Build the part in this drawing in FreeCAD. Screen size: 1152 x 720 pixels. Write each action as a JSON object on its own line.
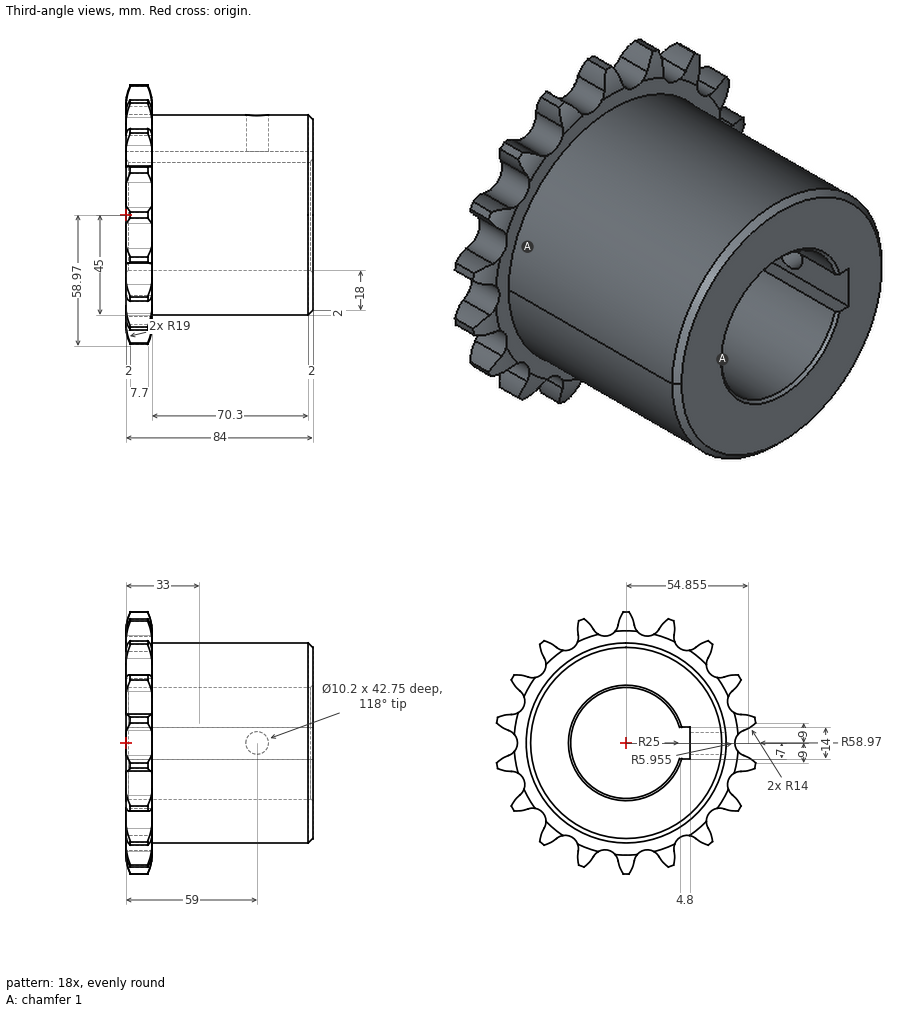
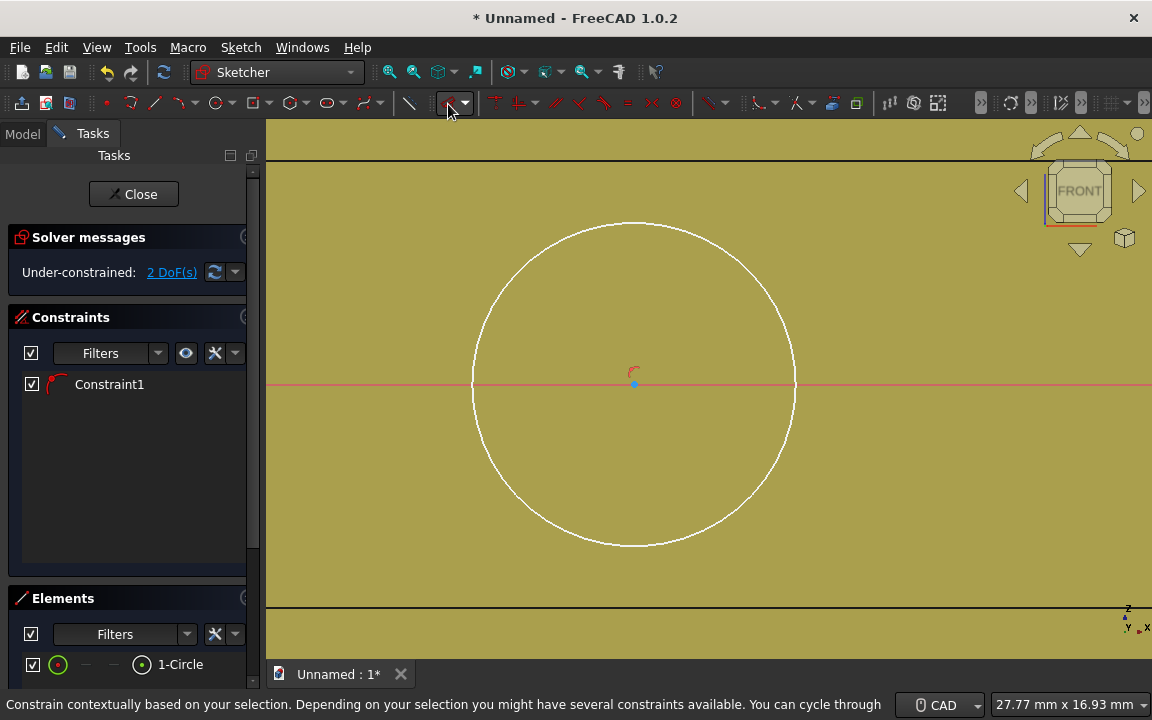
{"action": "left_click", "coordinate": [748, 270]}
{"action": "left_click", "coordinate": [771, 247]}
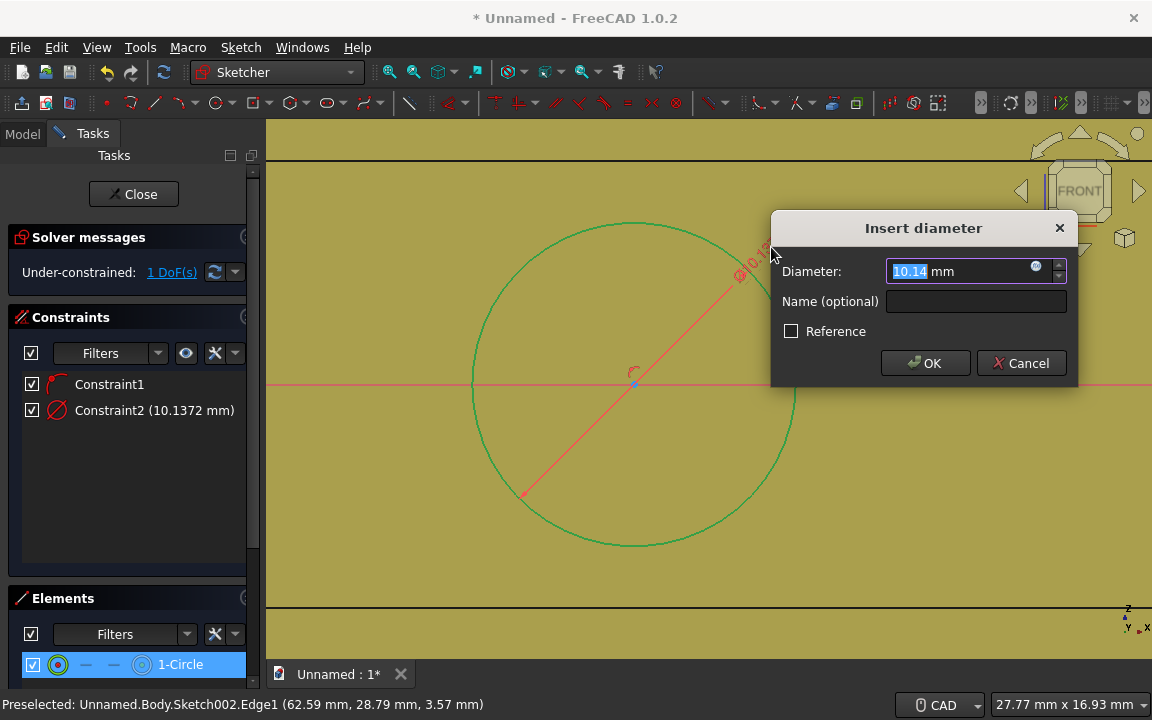
{"action": "type", "text": "10.2"}
{"action": "key", "text": "Return"}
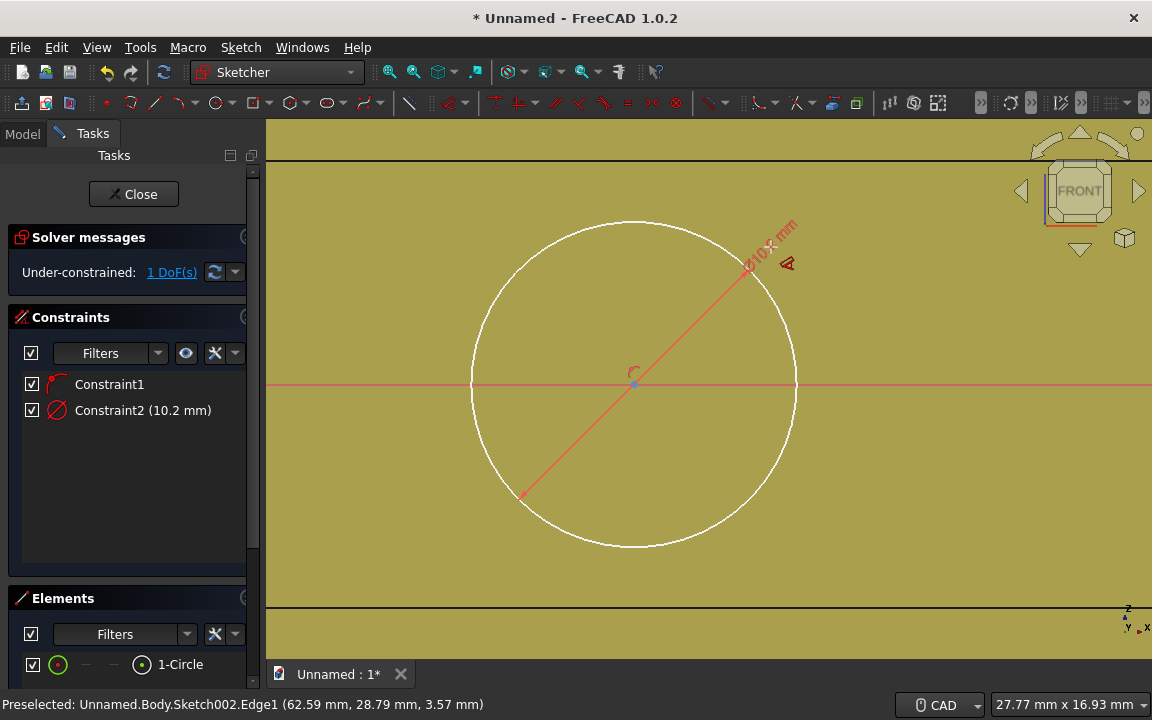
{"action": "left_click", "coordinate": [634, 385]}
{"action": "left_click", "coordinate": [386, 419]}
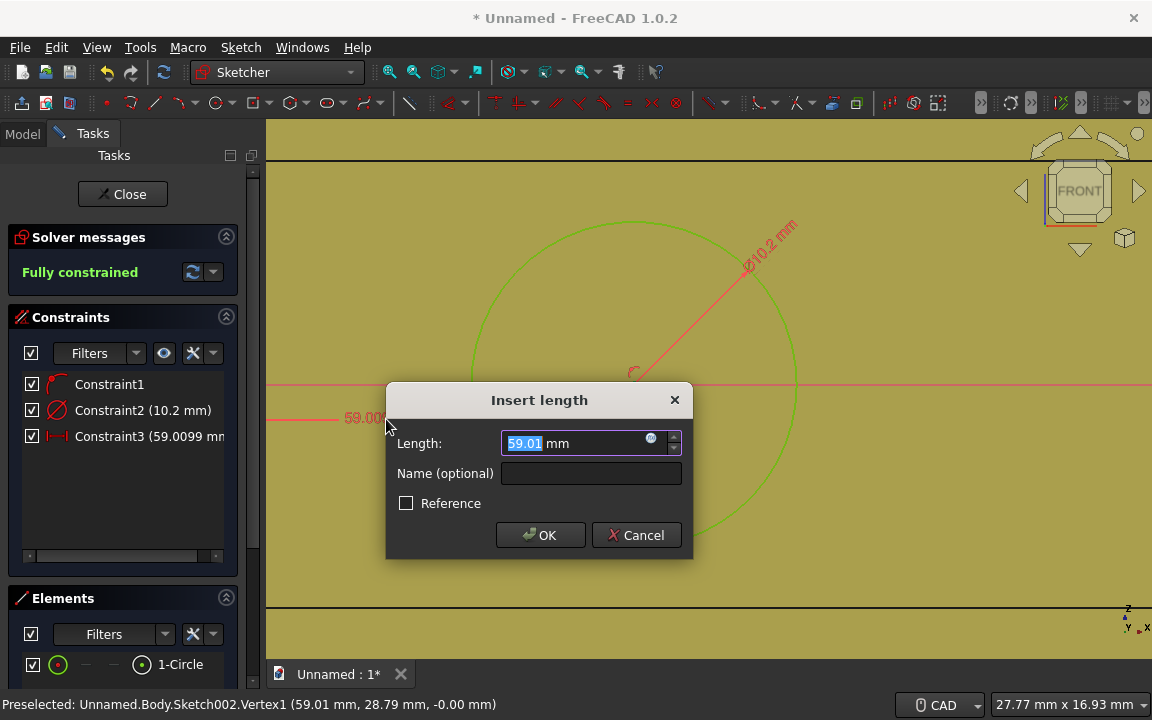
{"action": "type", "text": "59"}
{"action": "key", "text": "Return"}
{"action": "key", "text": "Escape"}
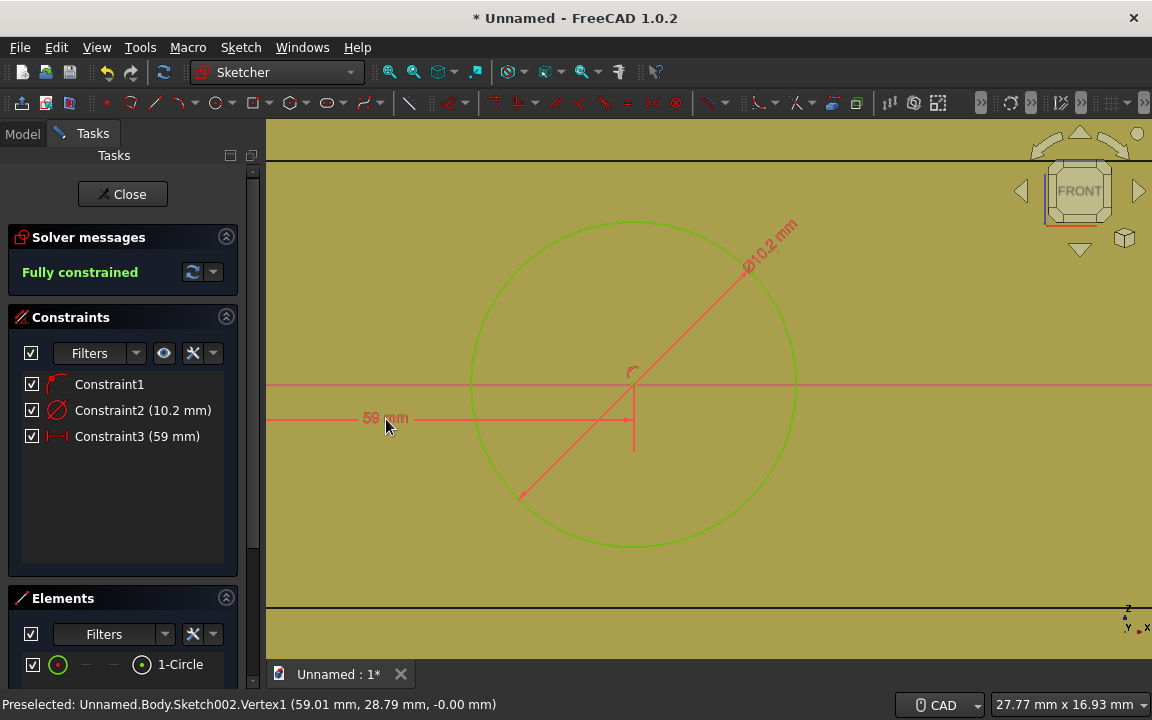
{"action": "left_click", "coordinate": [123, 194]}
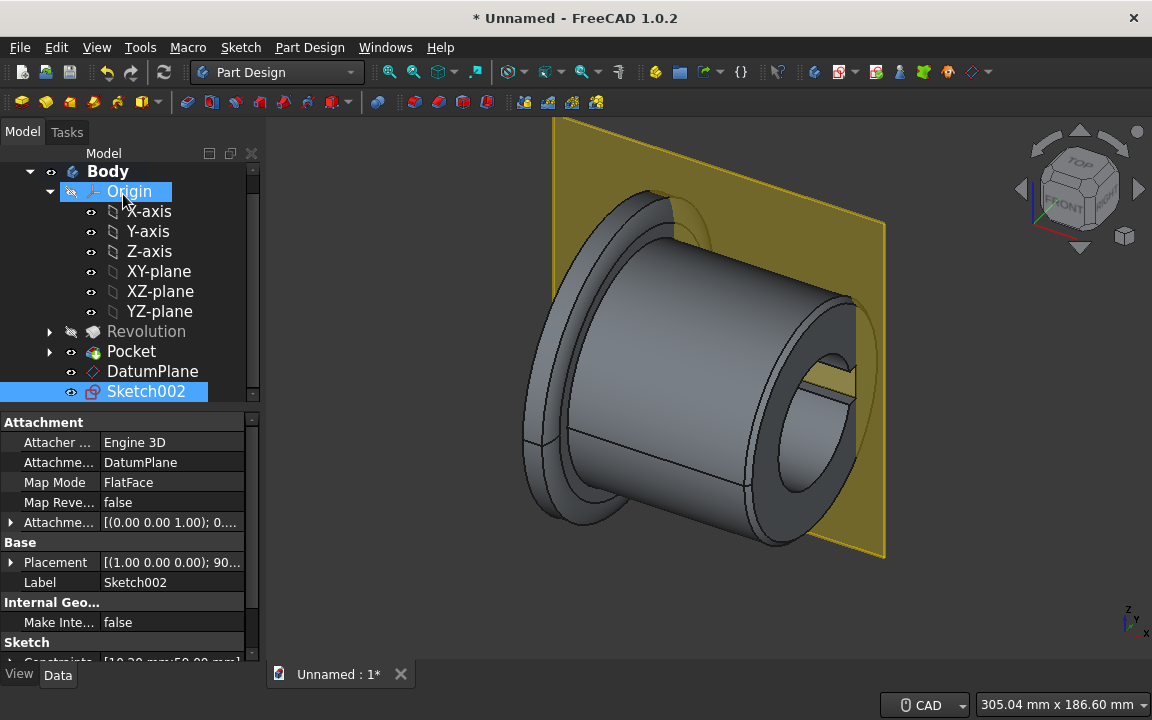
{"action": "left_click", "coordinate": [212, 102]}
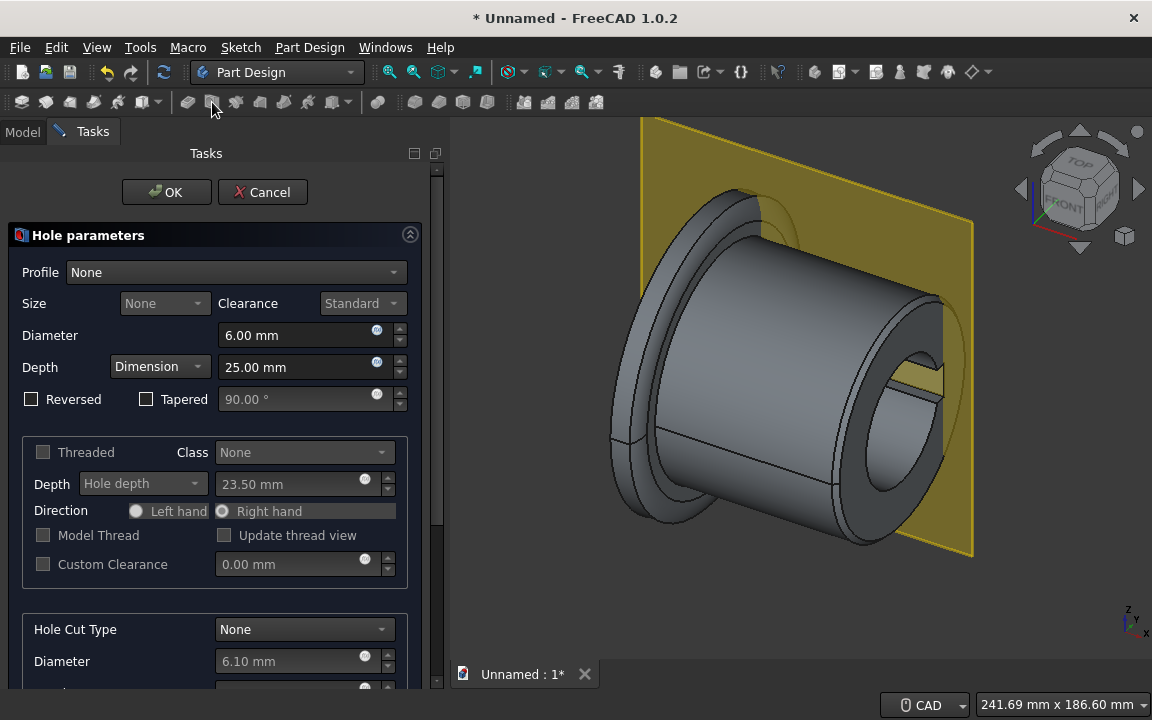
{"action": "triple_click", "coordinate": [305, 335]}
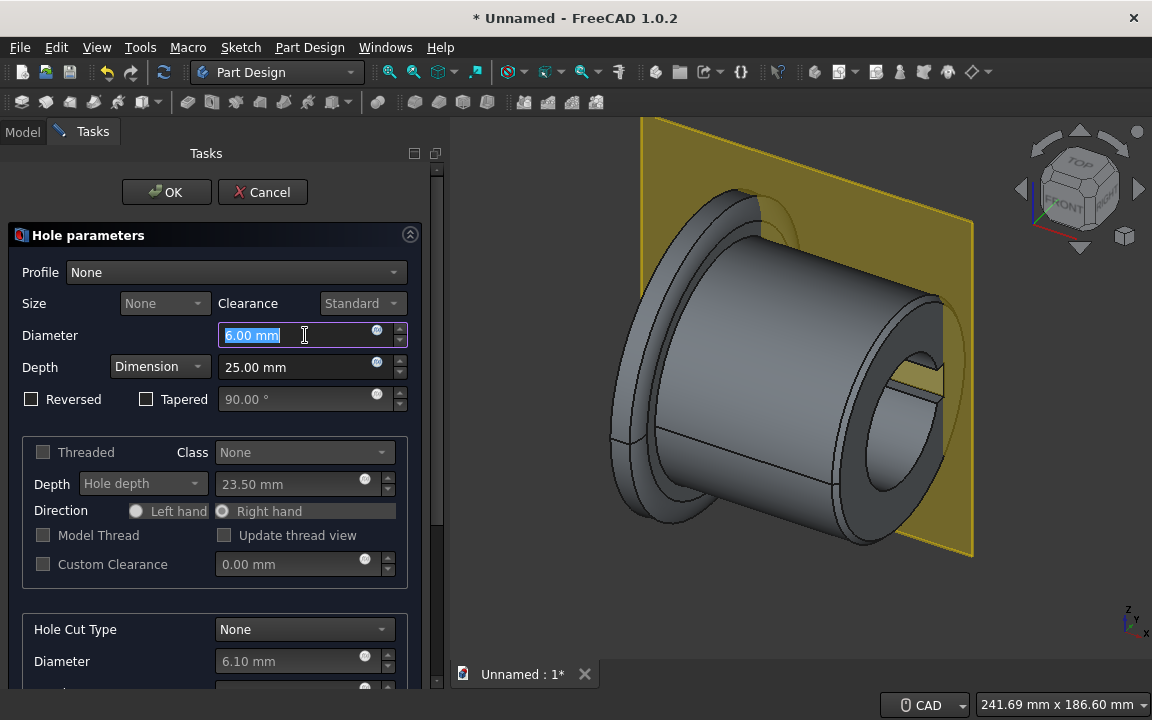
{"action": "type", "text": "10.2"}
{"action": "key", "text": "Tab"}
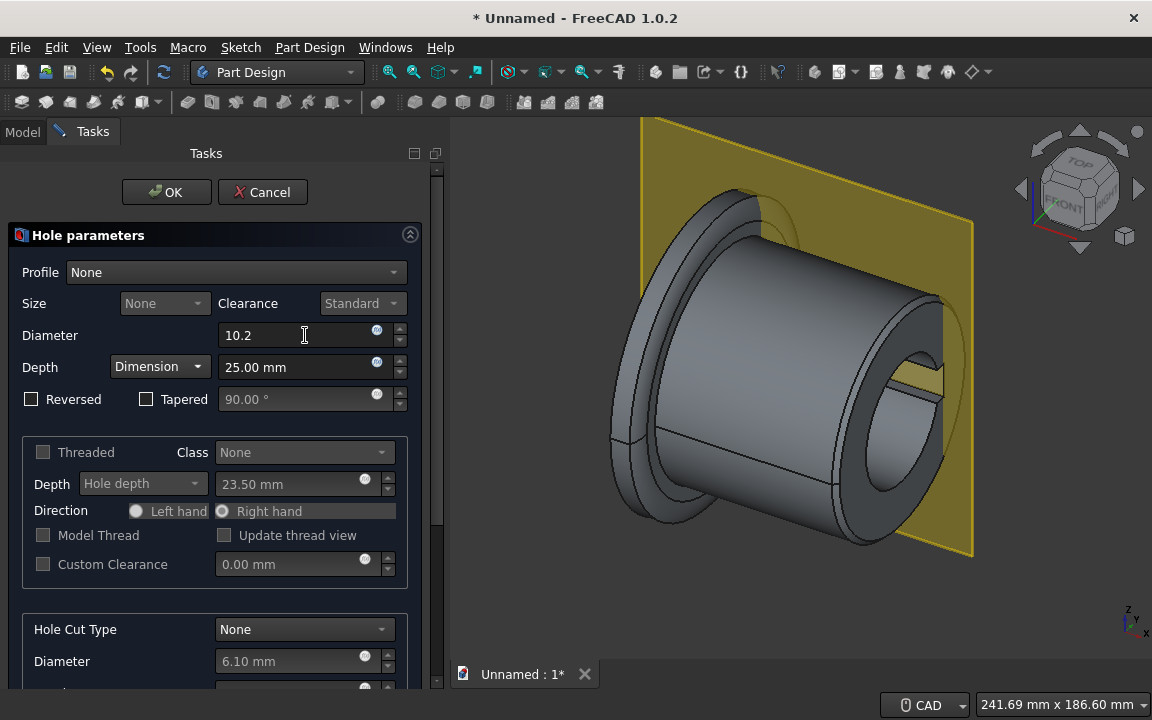
{"action": "triple_click", "coordinate": [305, 367]}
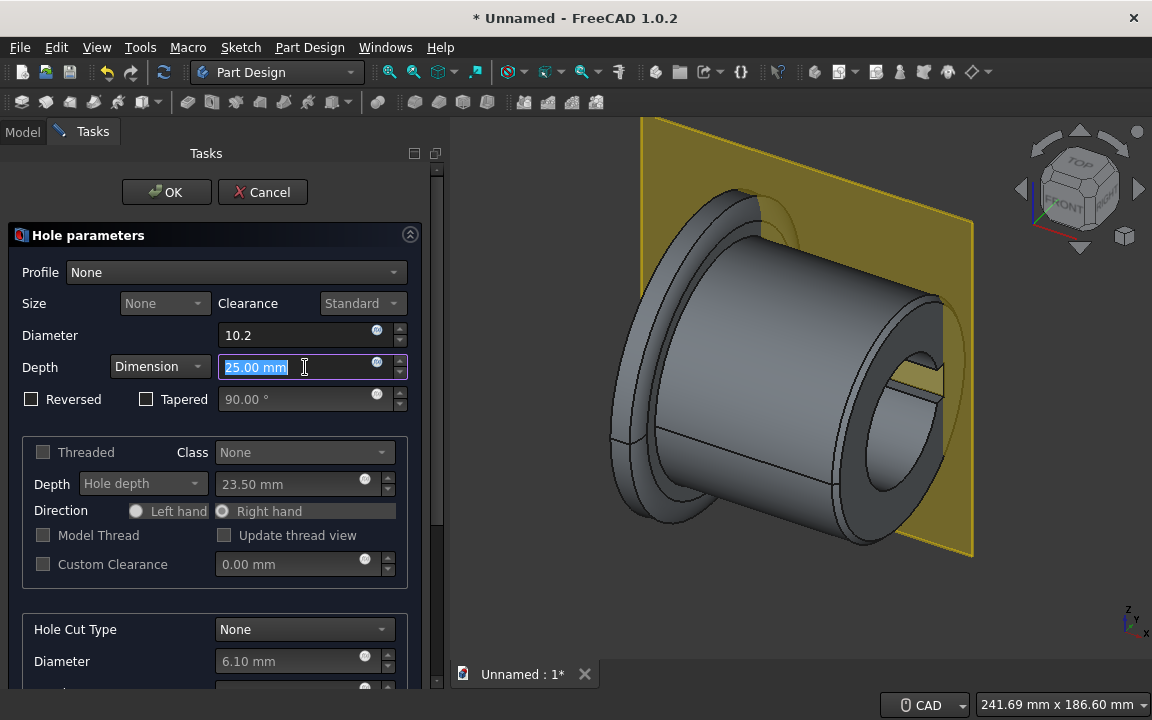
{"action": "type", "text": "42.75"}
{"action": "key", "text": "Tab"}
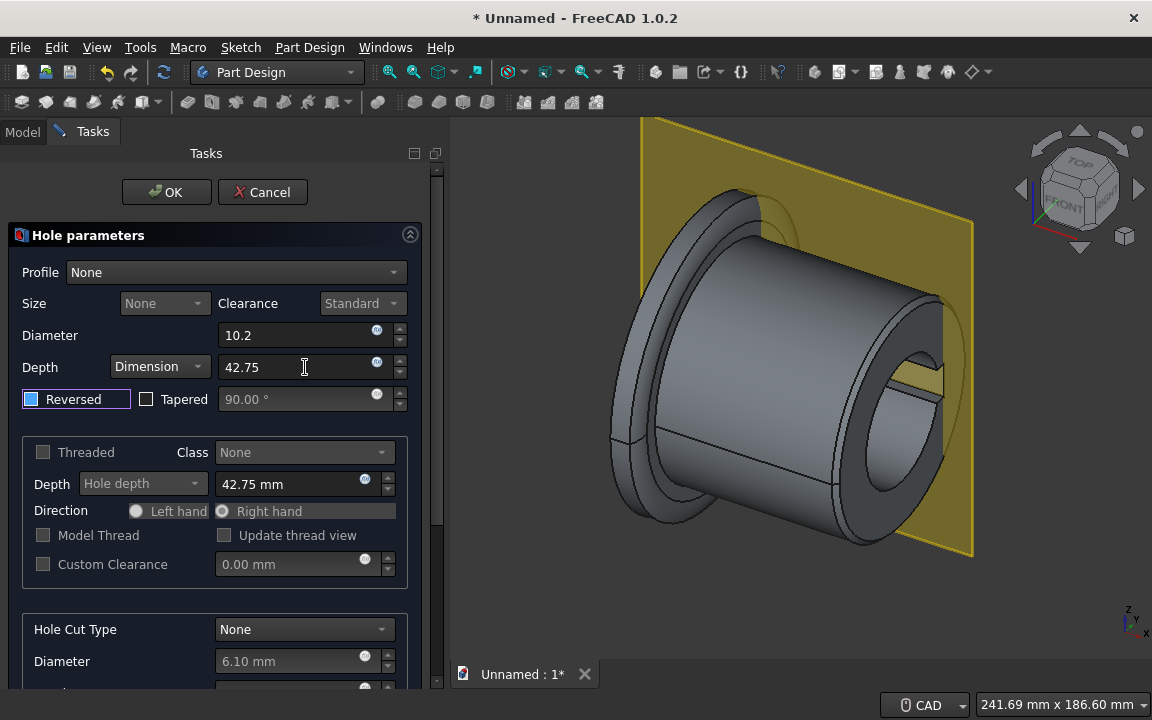
{"action": "left_click", "coordinate": [167, 192]}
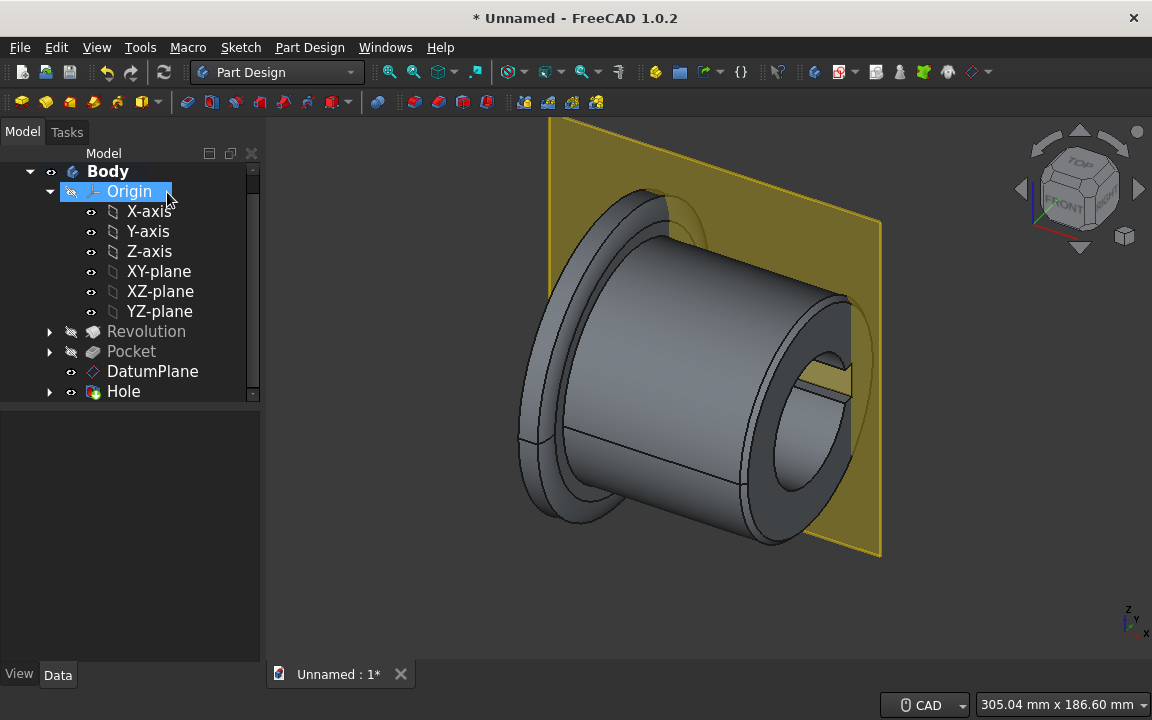
{"action": "left_click", "coordinate": [116, 372]}
{"action": "key", "text": "space"}